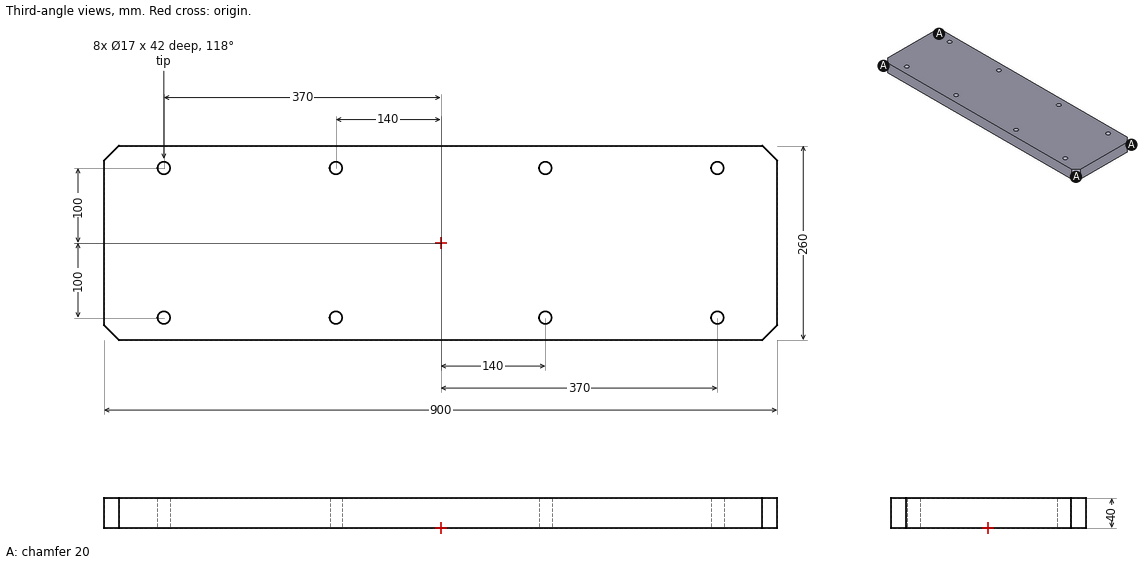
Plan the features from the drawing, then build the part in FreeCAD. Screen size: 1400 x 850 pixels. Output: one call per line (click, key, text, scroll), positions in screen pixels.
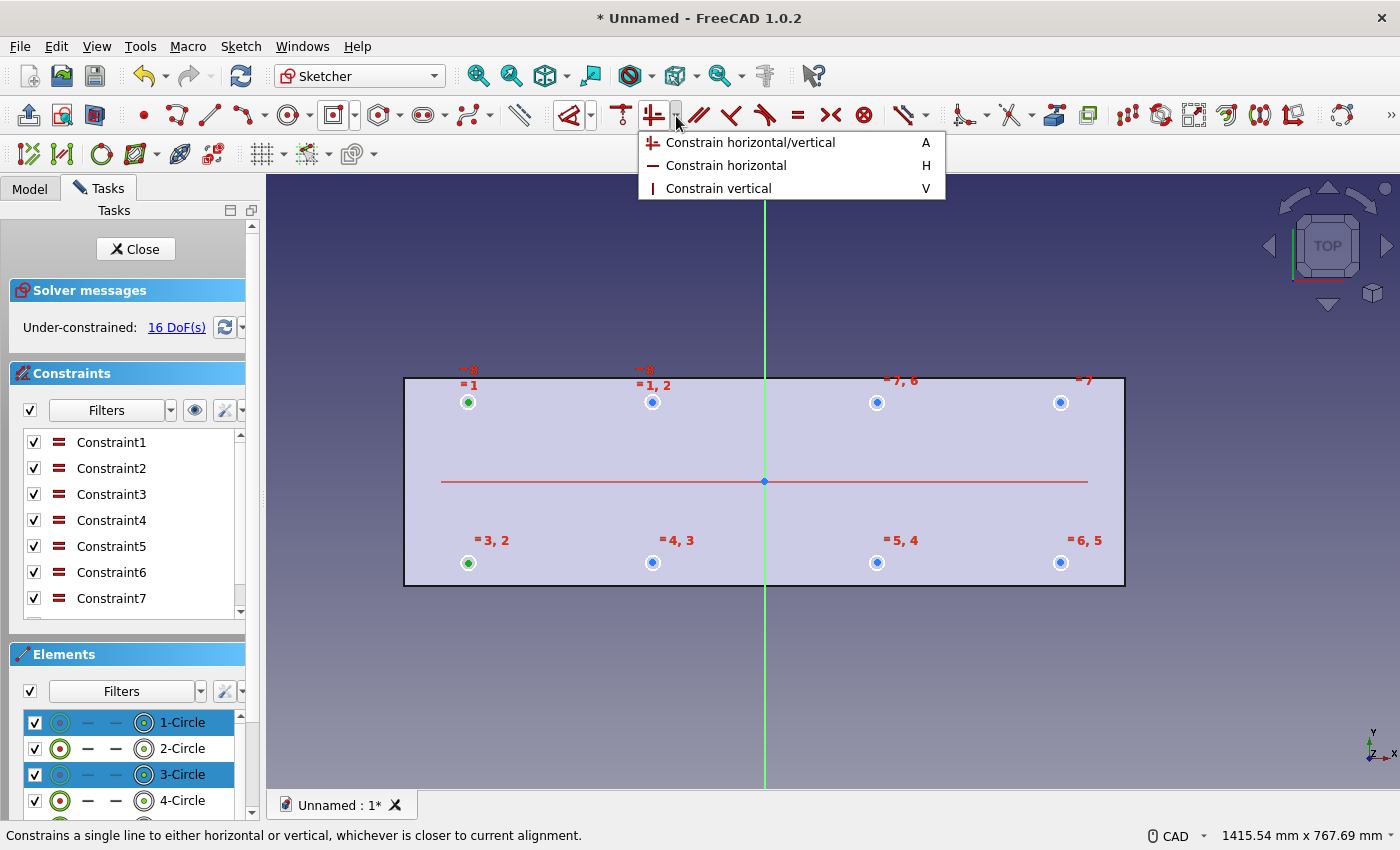
click(792, 188)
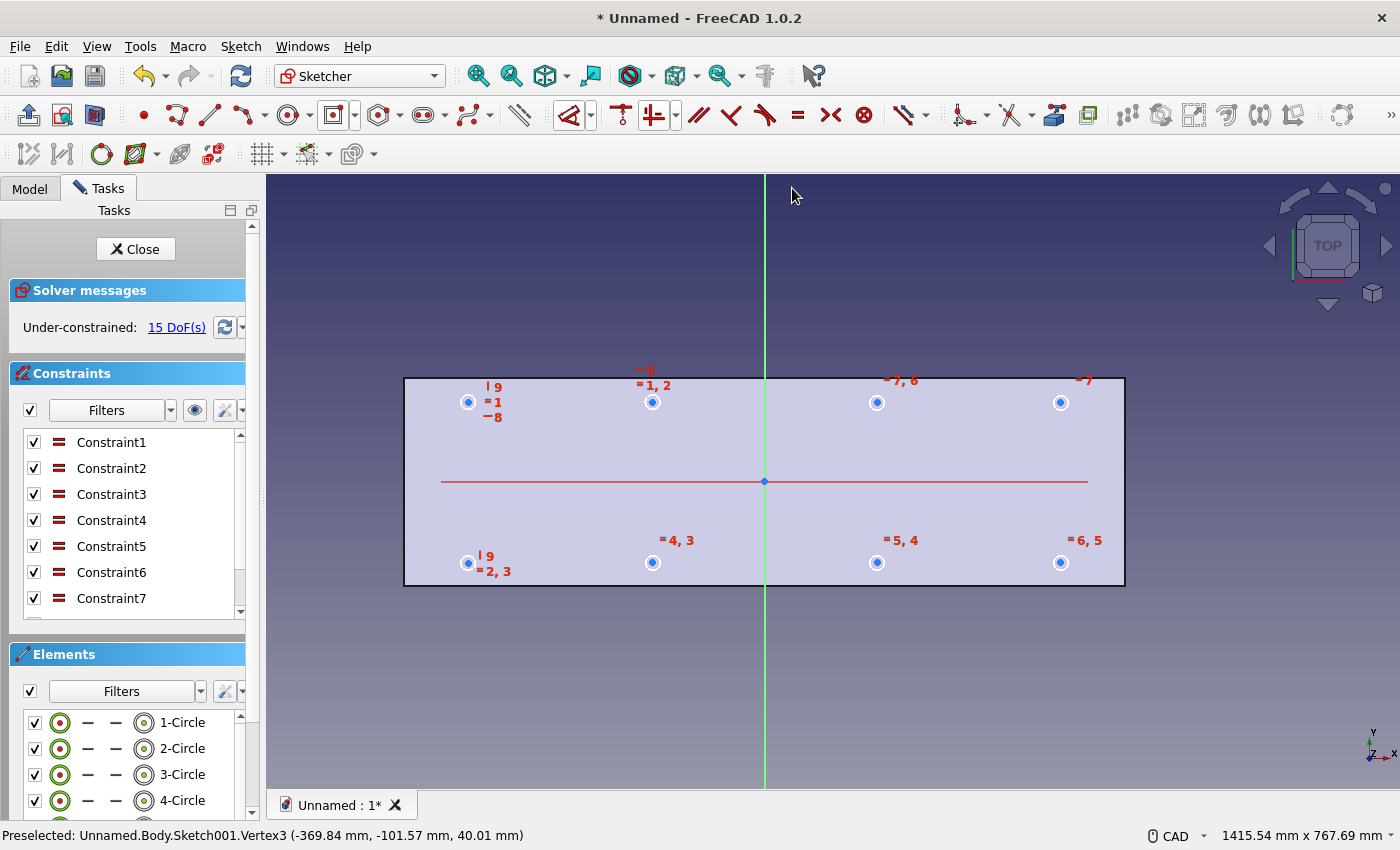
click(653, 402)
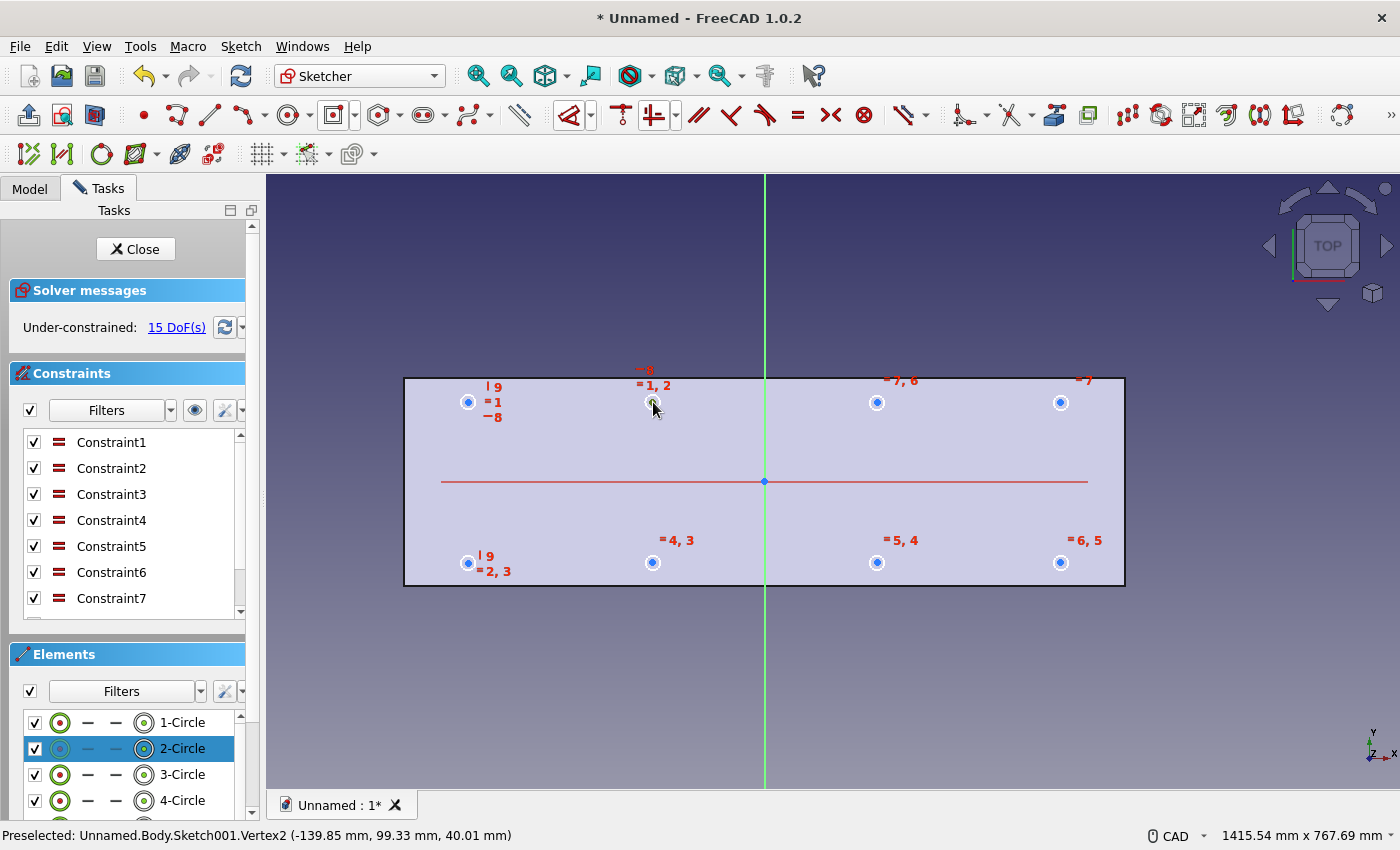
click(653, 563)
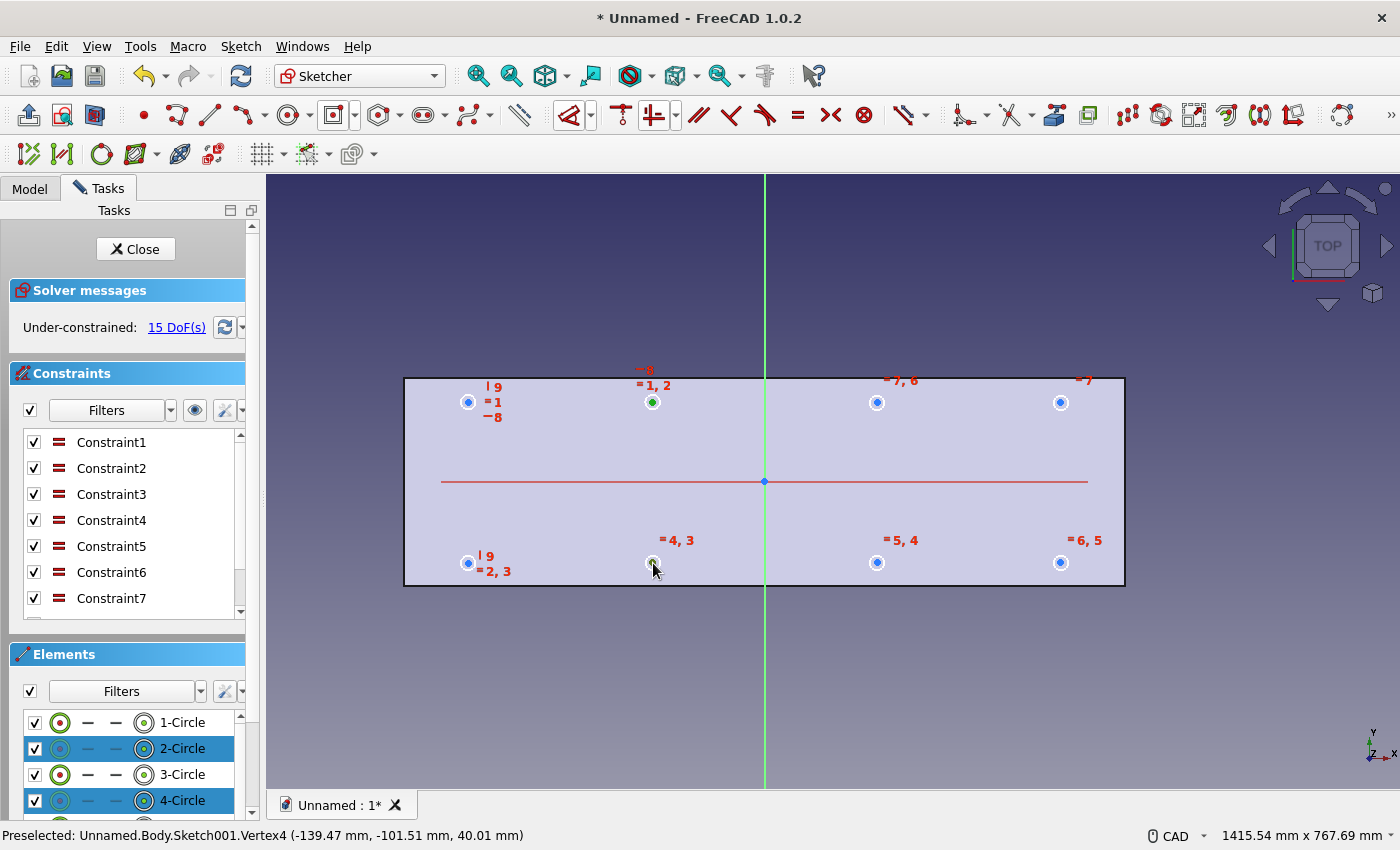
click(676, 116)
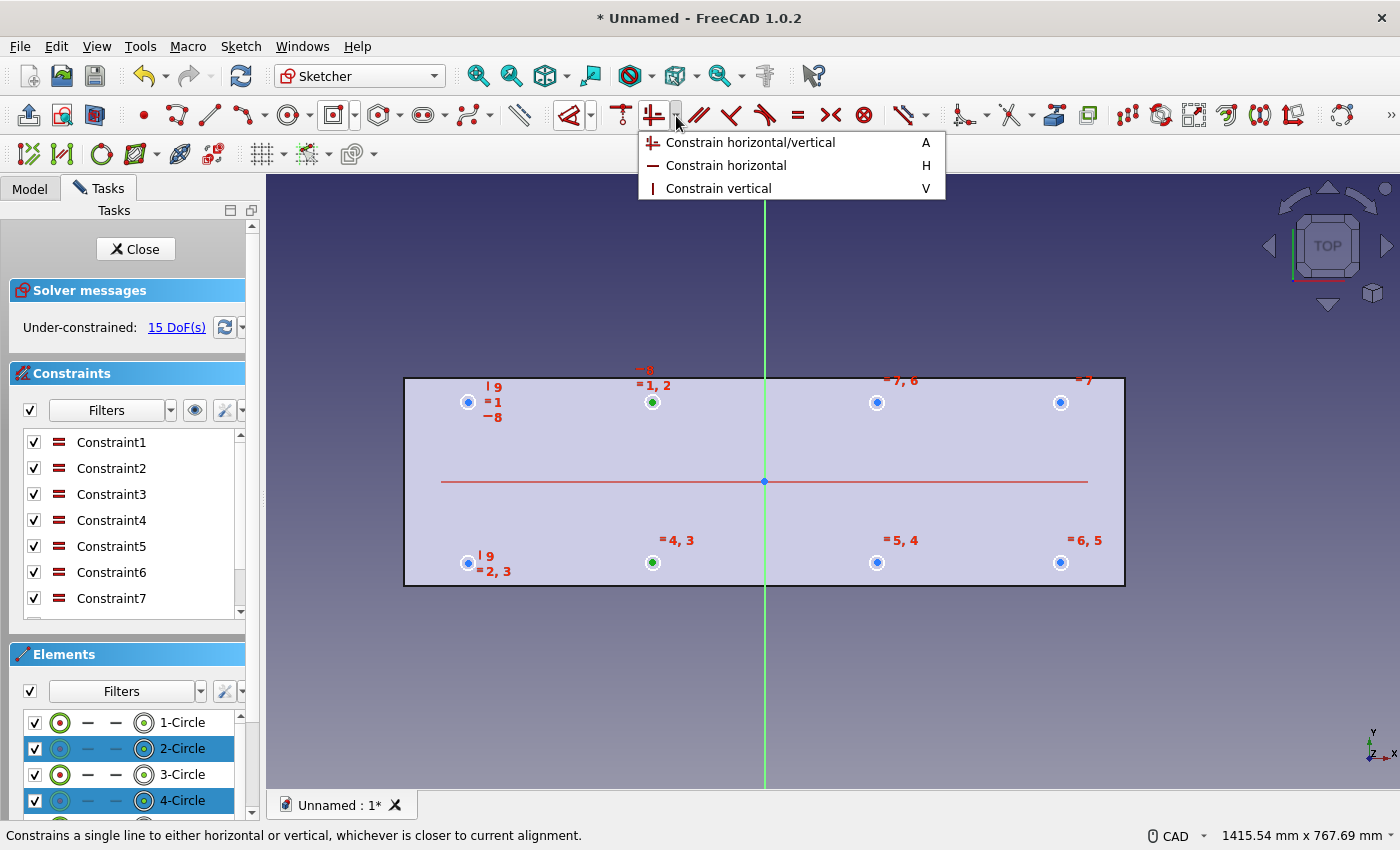
click(792, 188)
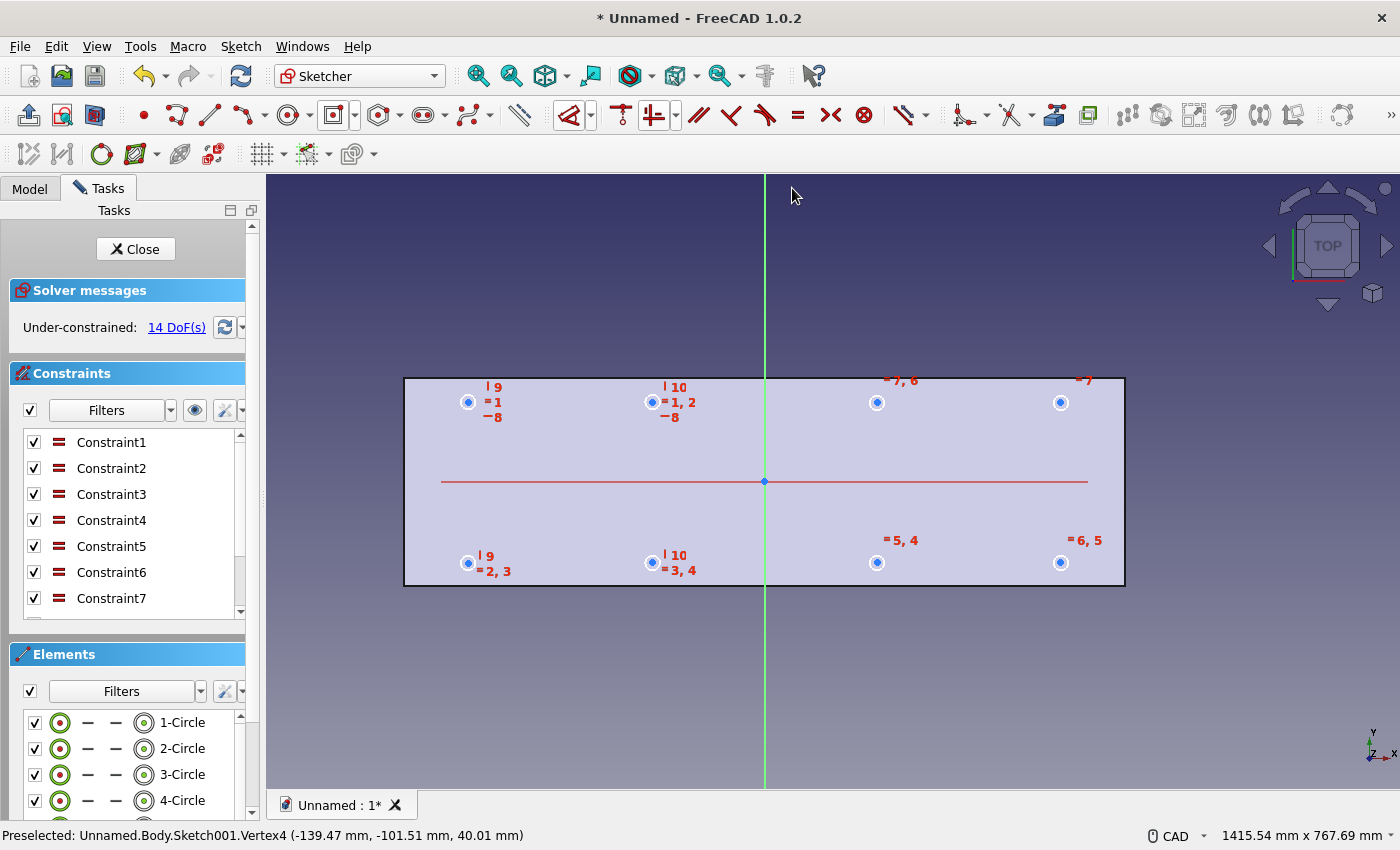
click(468, 563)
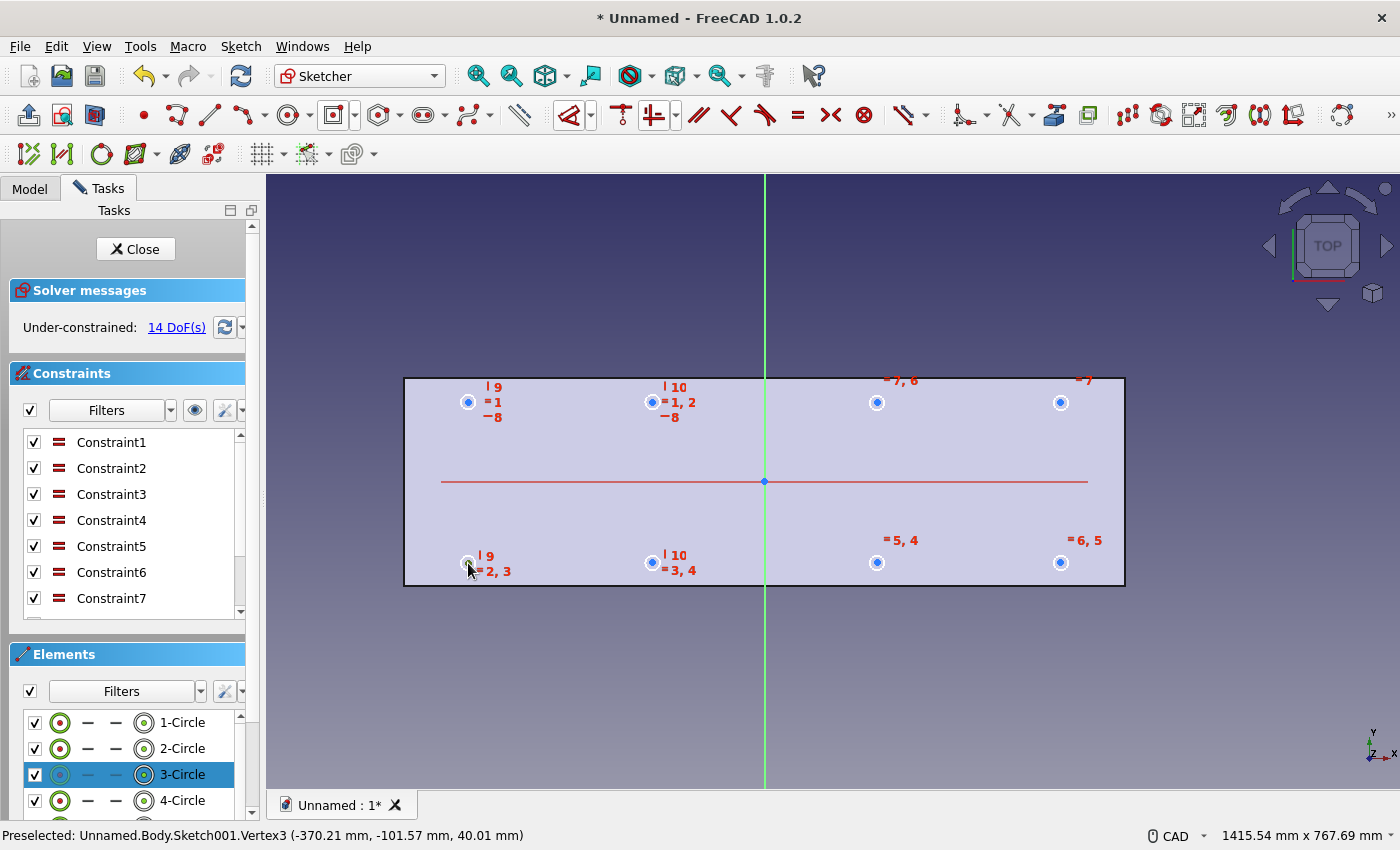
click(653, 563)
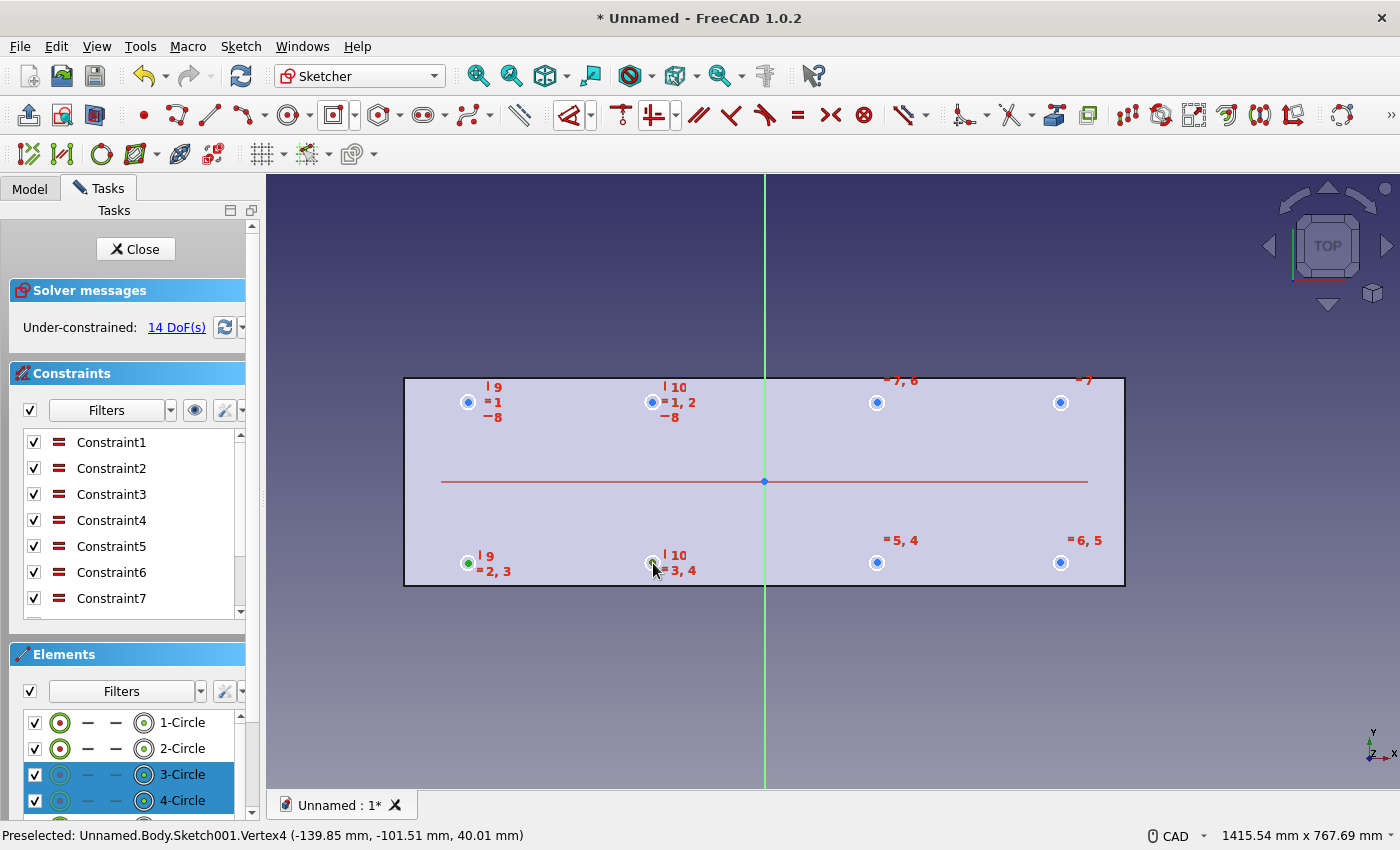
key(h)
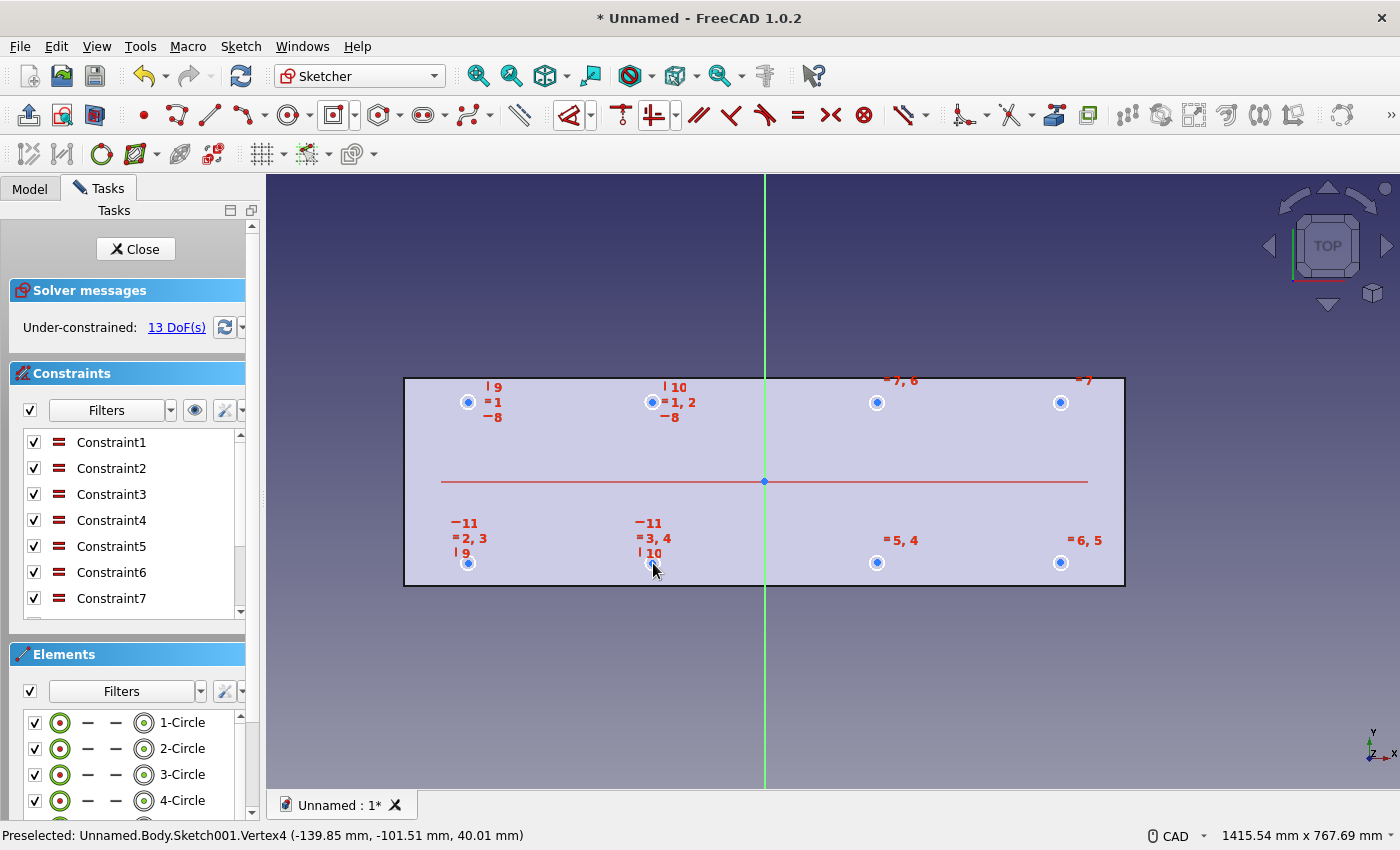
click(653, 563)